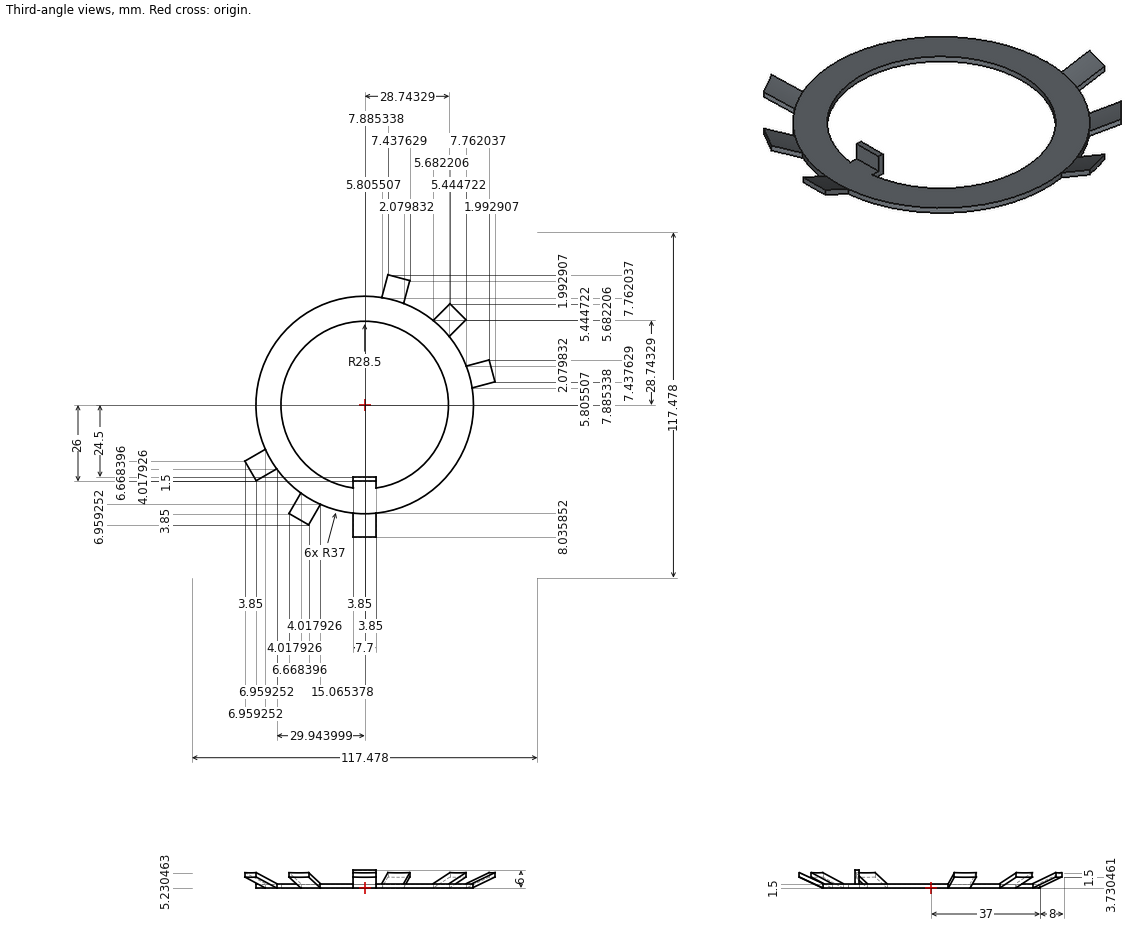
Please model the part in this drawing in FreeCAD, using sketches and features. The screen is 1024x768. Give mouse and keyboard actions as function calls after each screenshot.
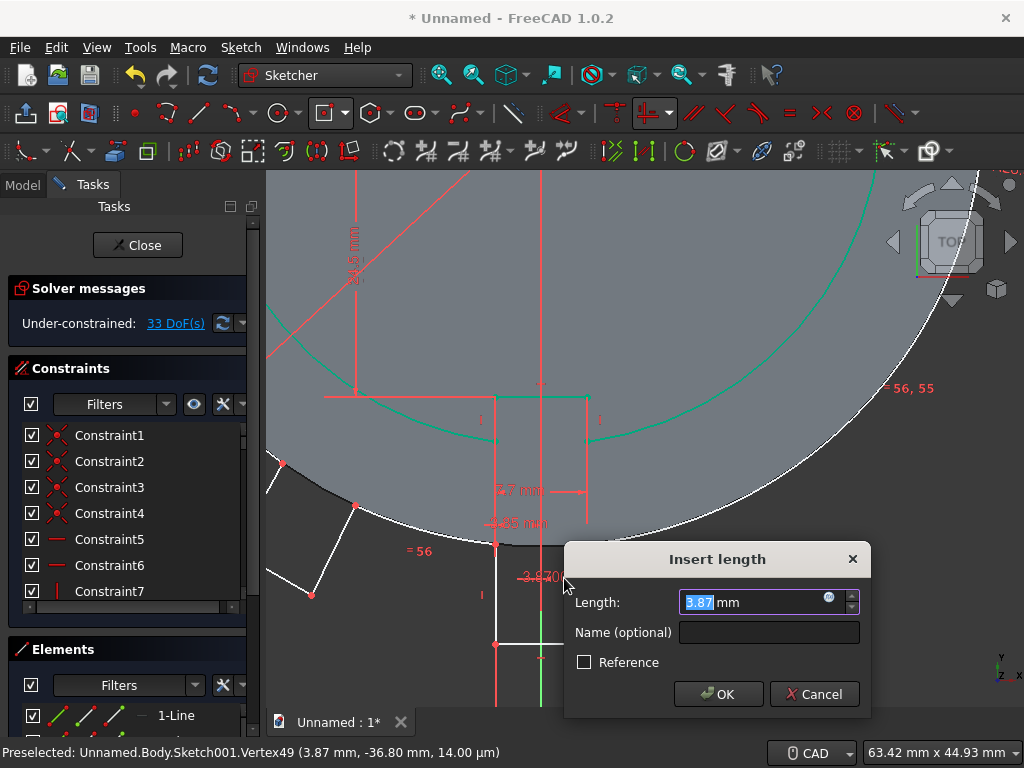
text(3.85)
key(Return)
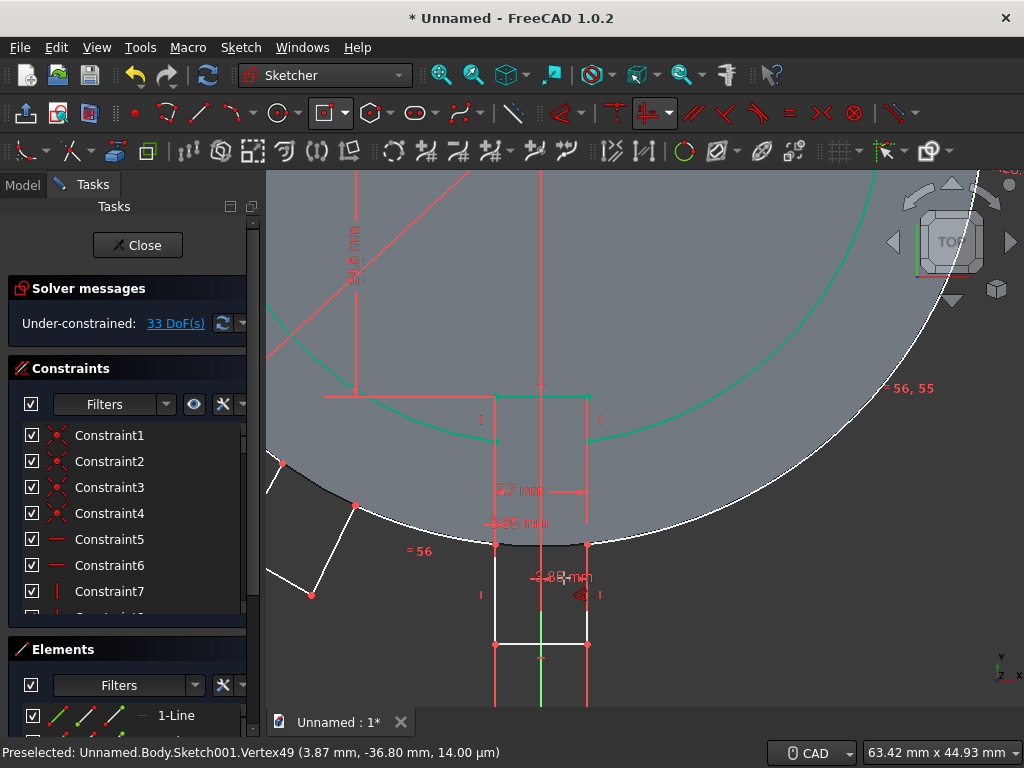
click(296, 586)
click(346, 573)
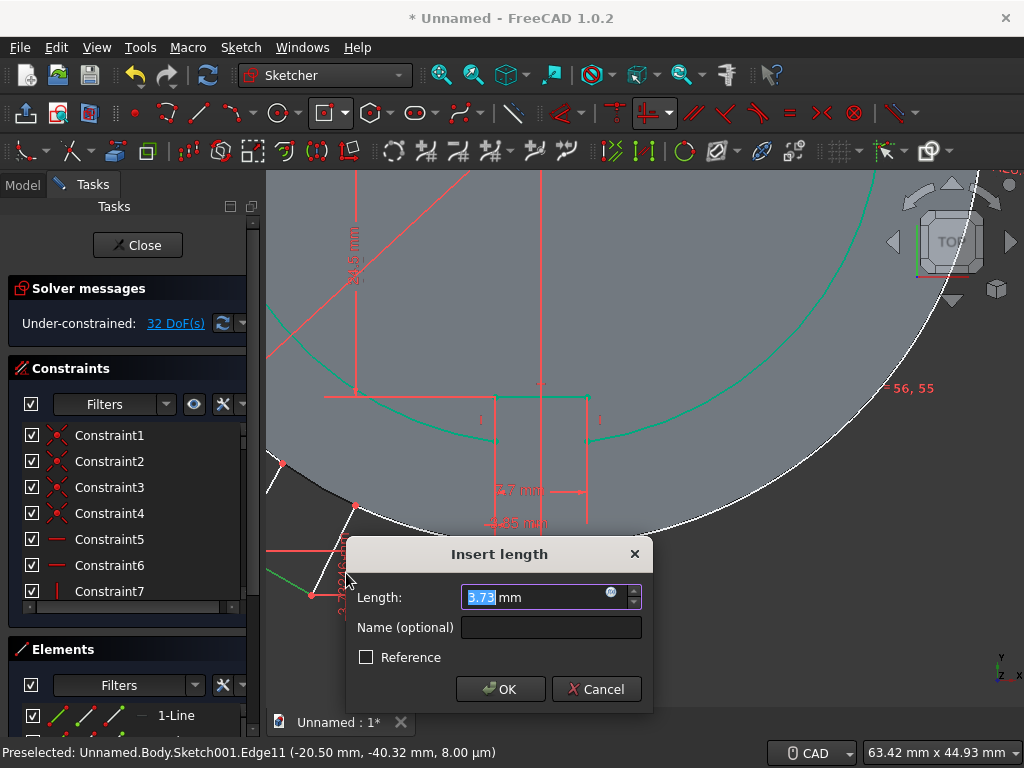
text(3.85)
key(Return)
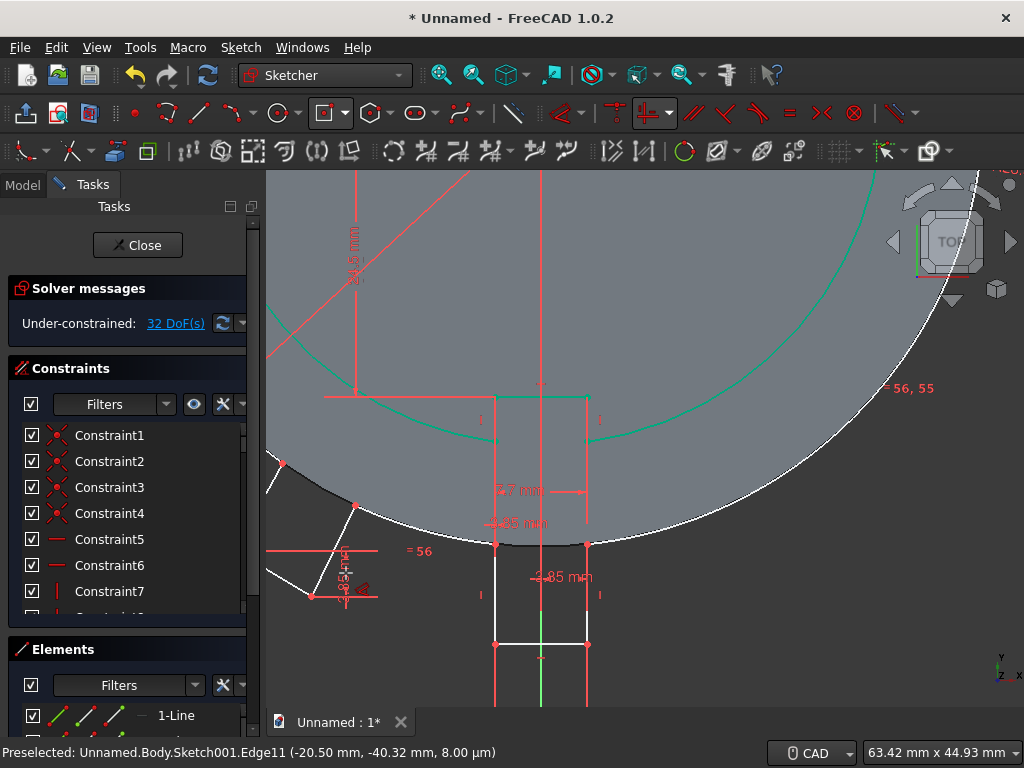
scroll(588, 548, down, 7)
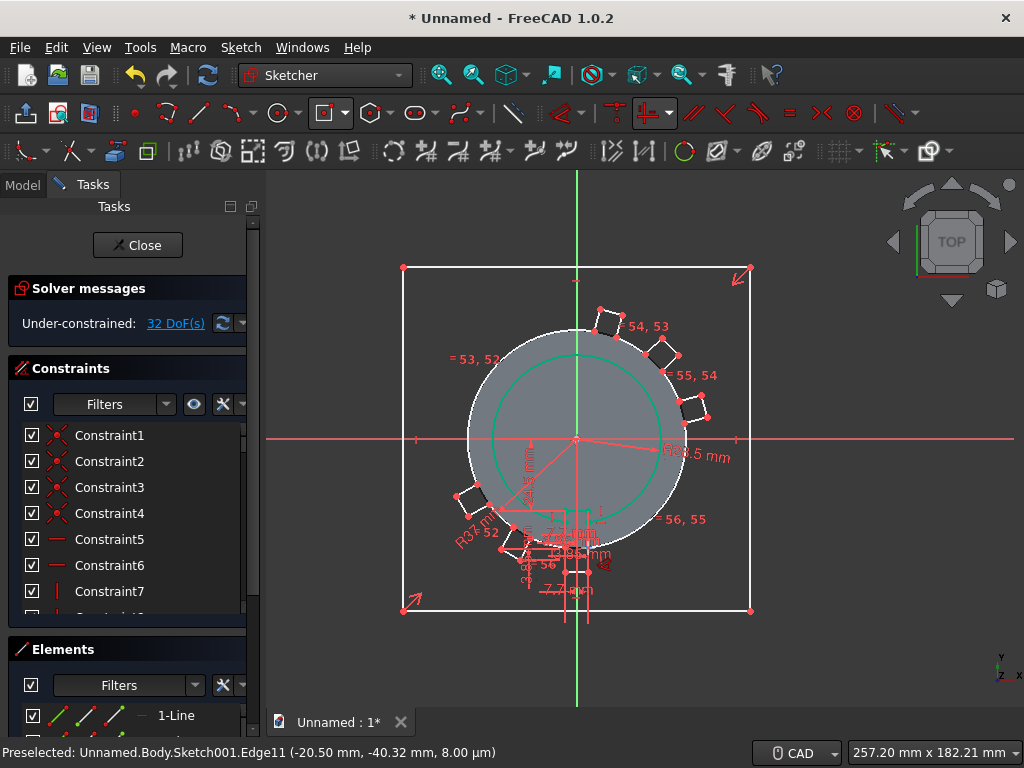
scroll(465, 510, up, 7)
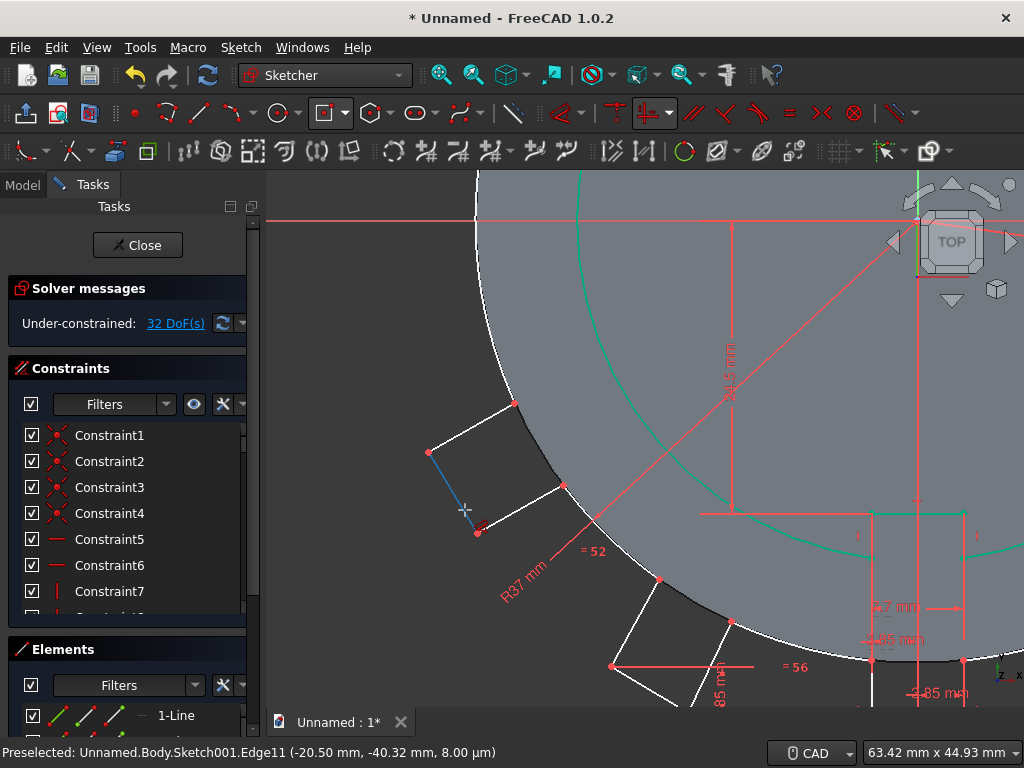
click(463, 509)
click(453, 567)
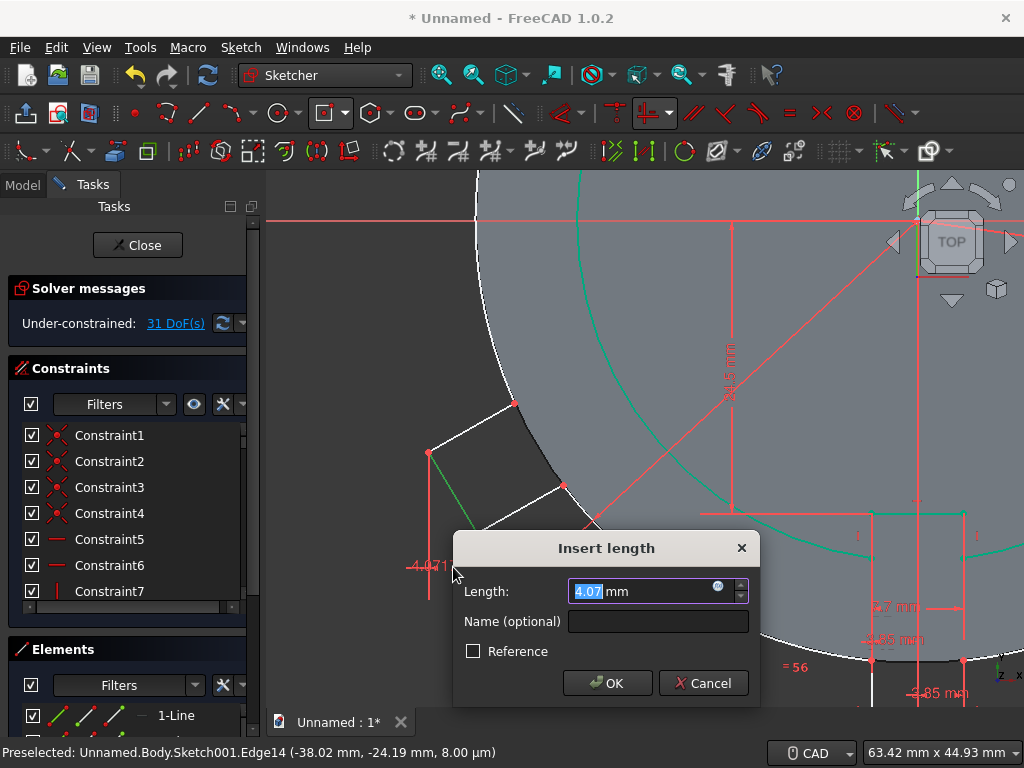
text(3.85)
key(Return)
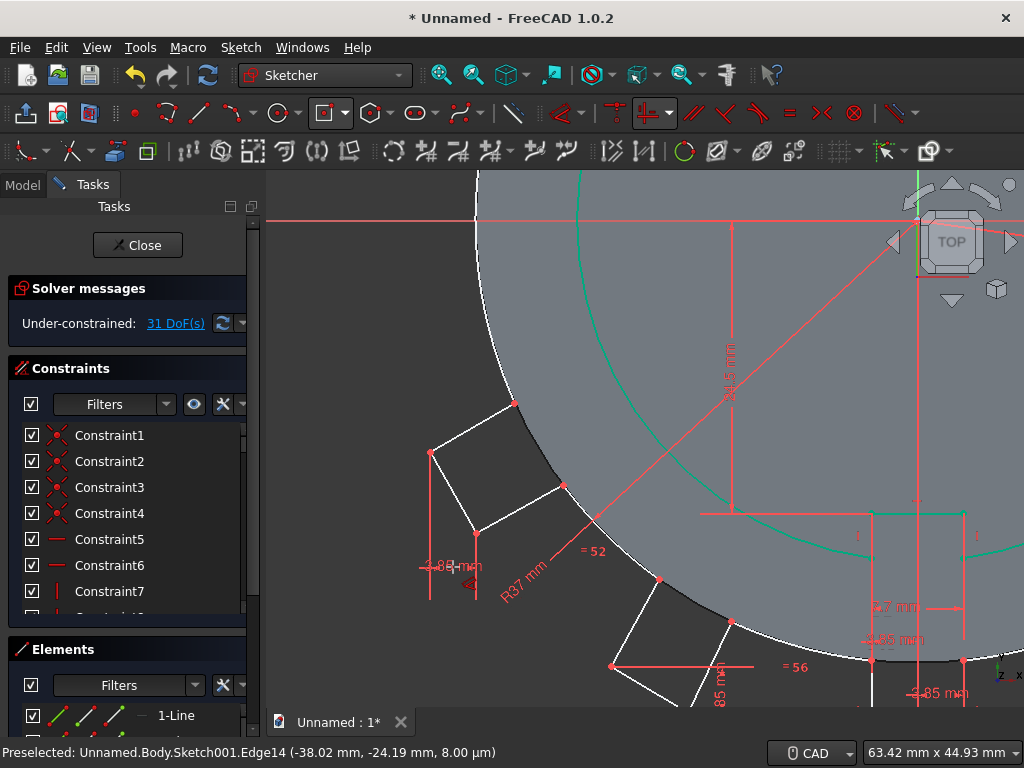
scroll(465, 510, down, 7)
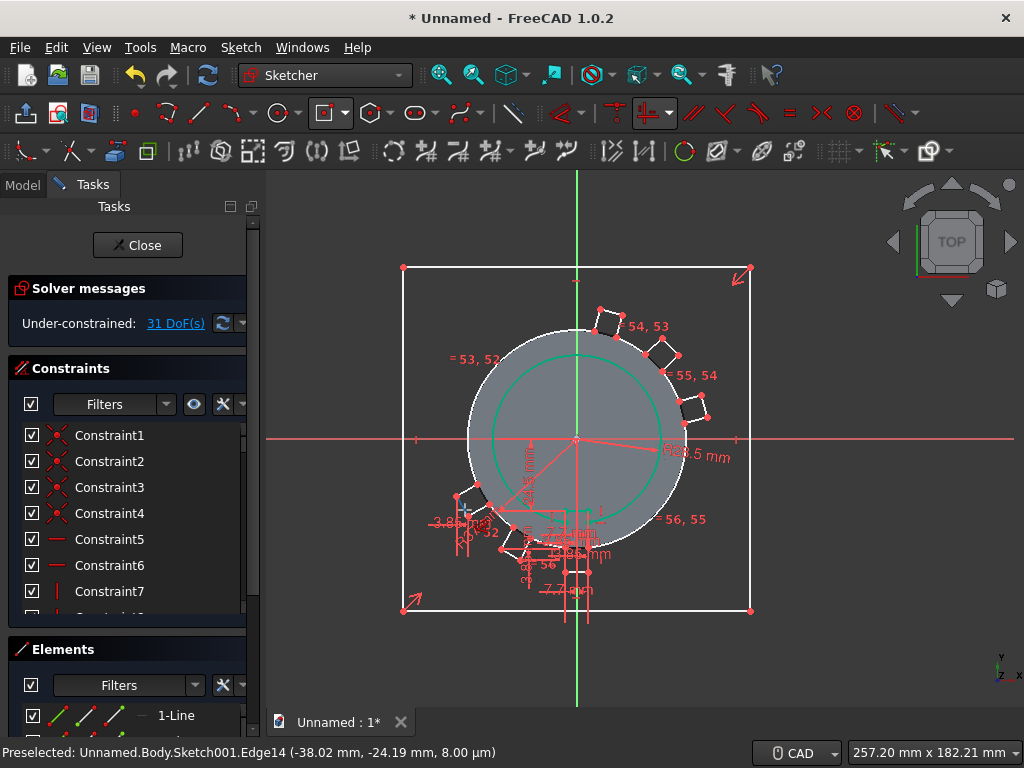
click(507, 611)
click(497, 645)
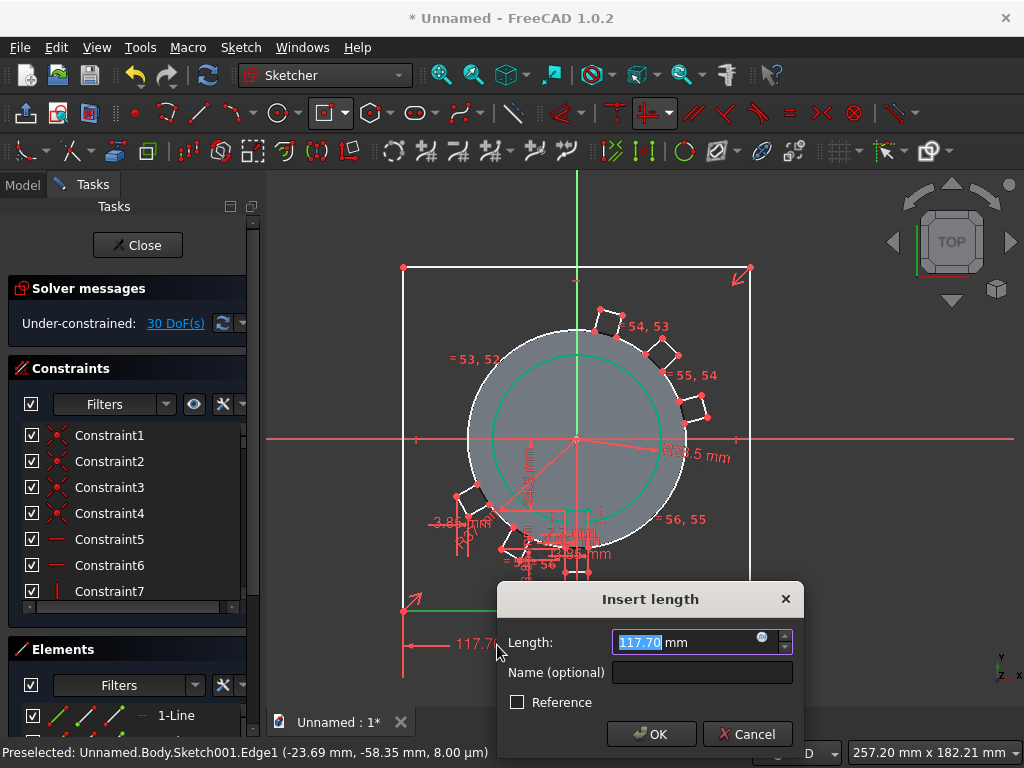
text(117.478)
key(Return)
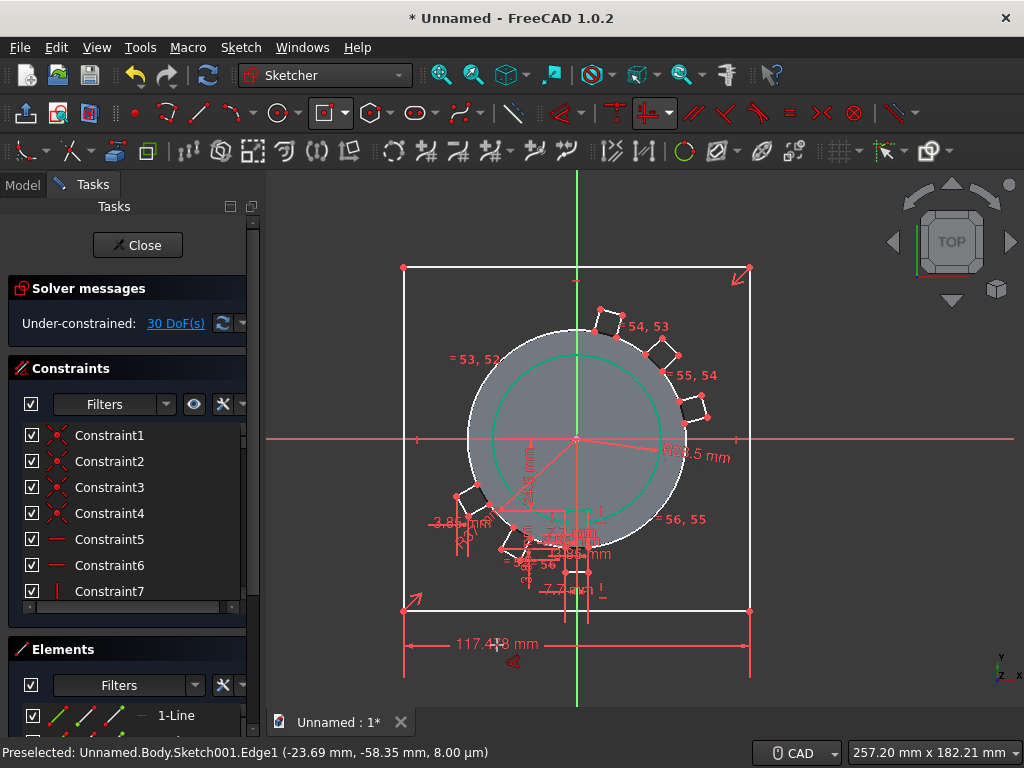
click(750, 508)
click(784, 360)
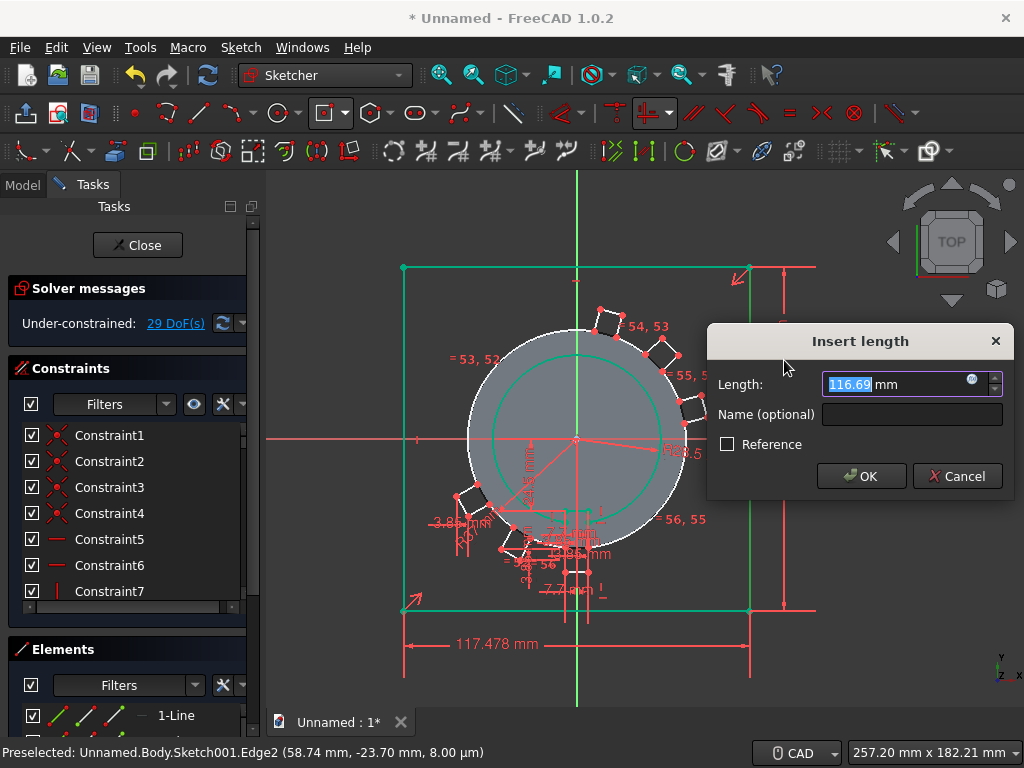
text(117.478)
key(Return)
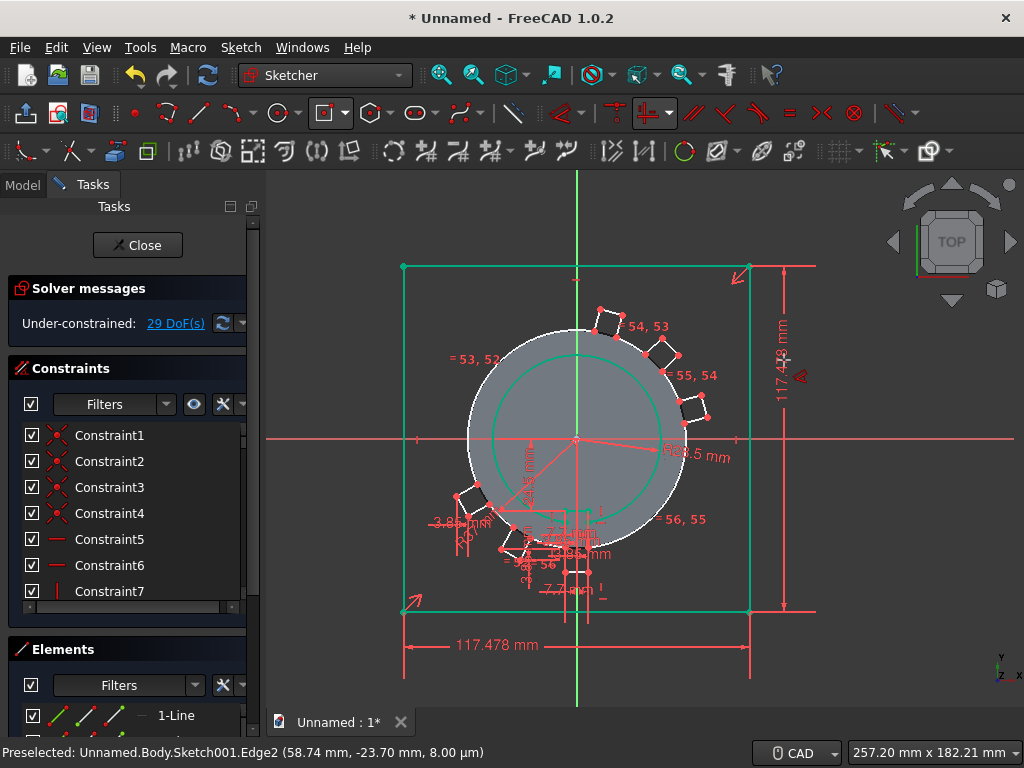
scroll(588, 557, up, 3)